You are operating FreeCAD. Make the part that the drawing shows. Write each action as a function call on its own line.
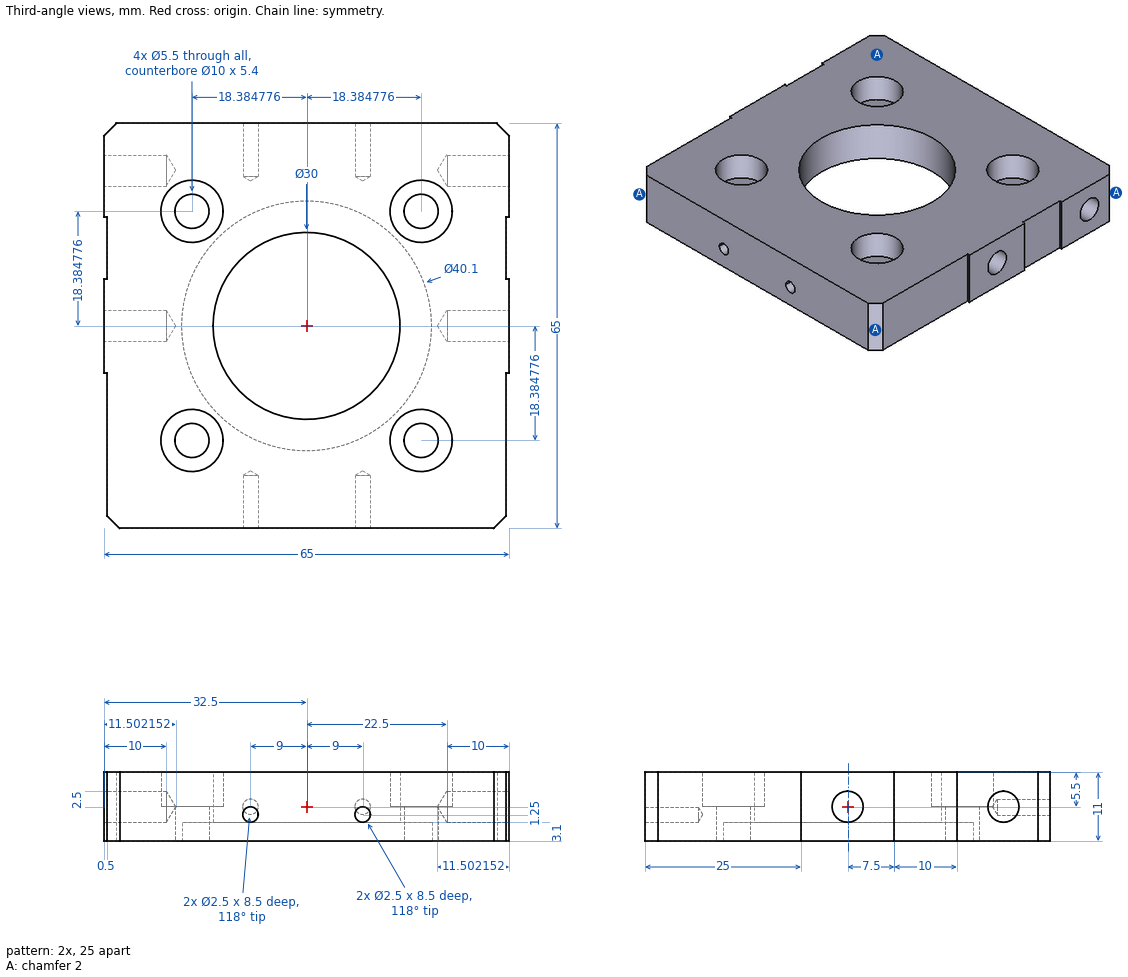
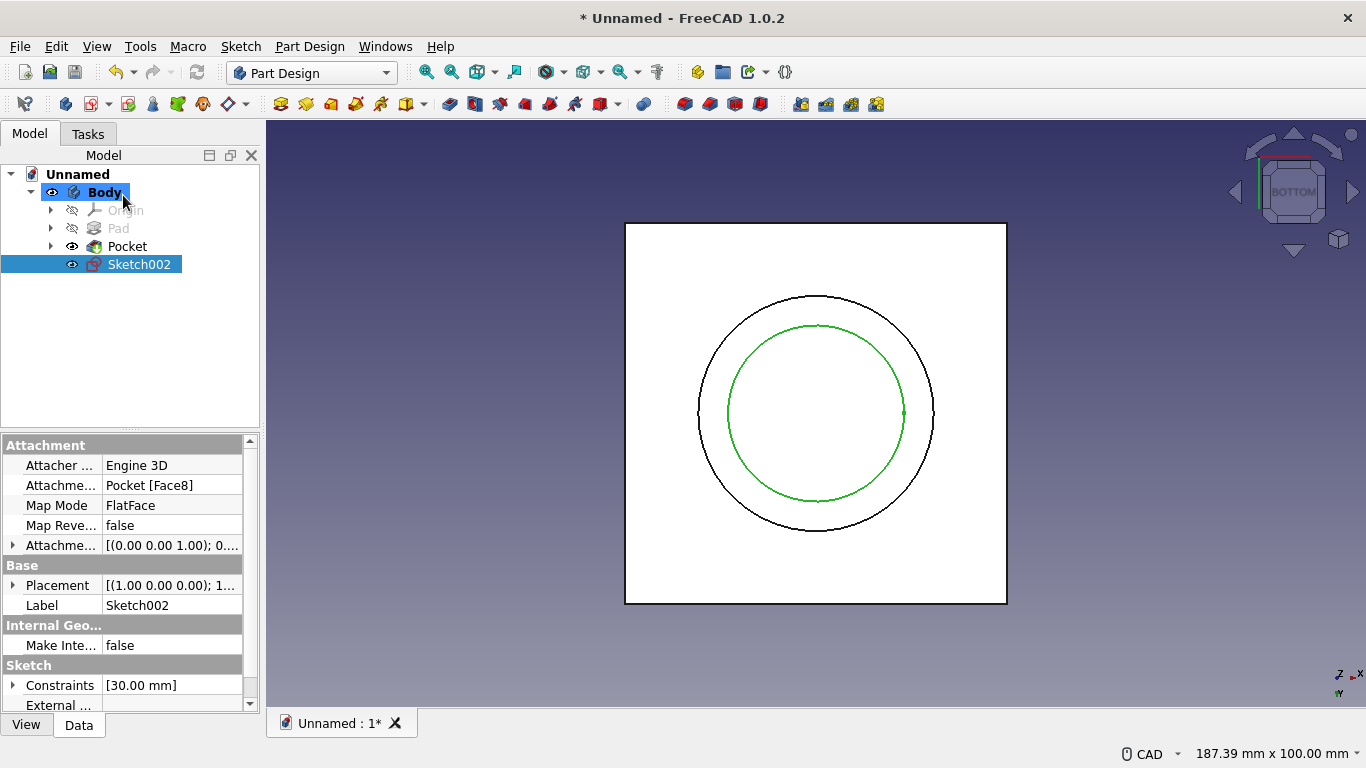
click(450, 104)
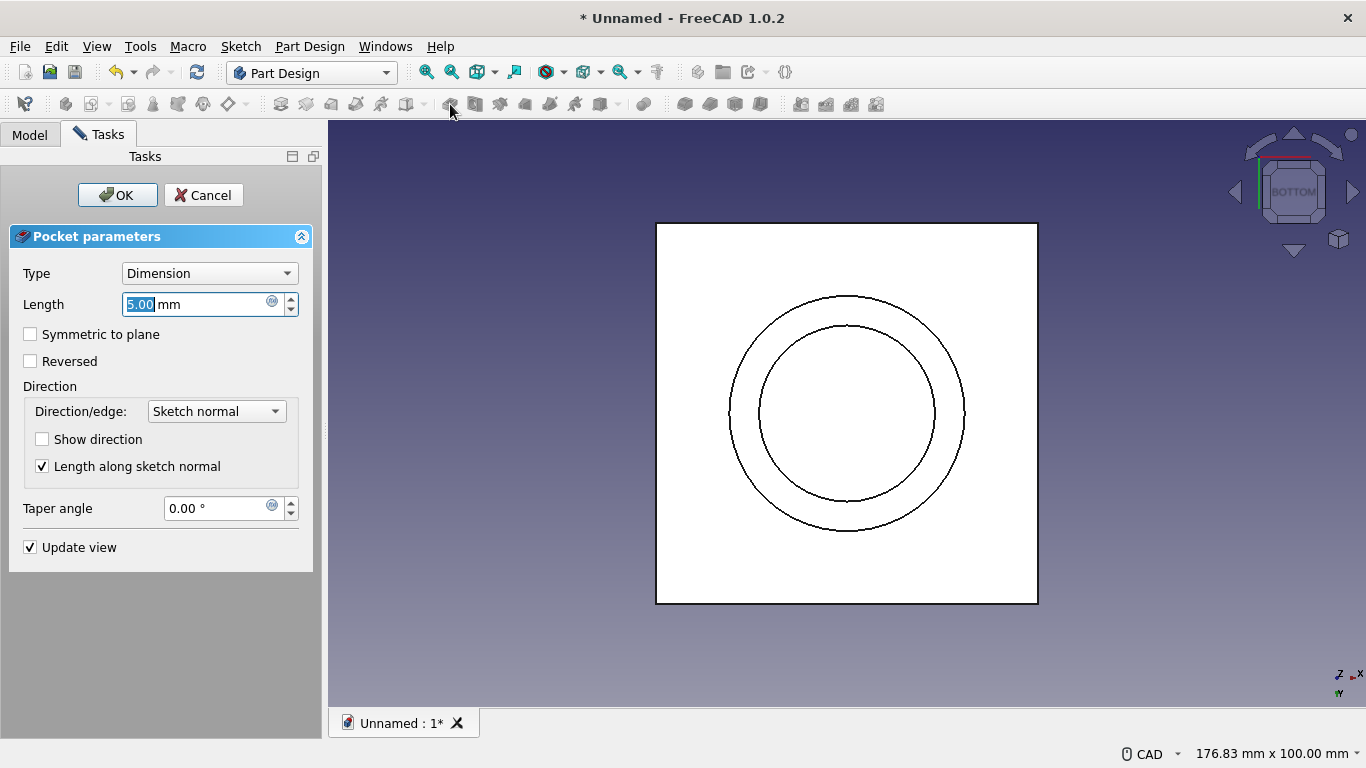
click(210, 274)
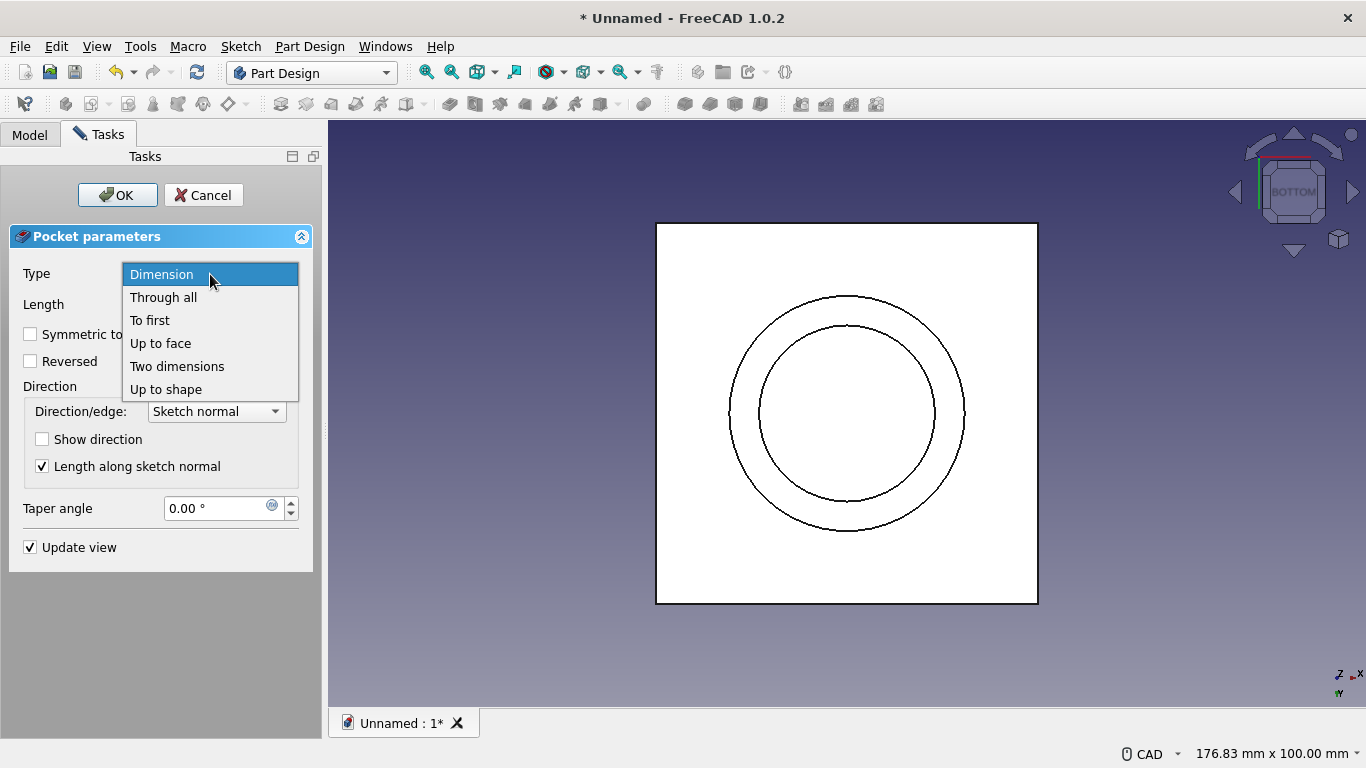
click(208, 298)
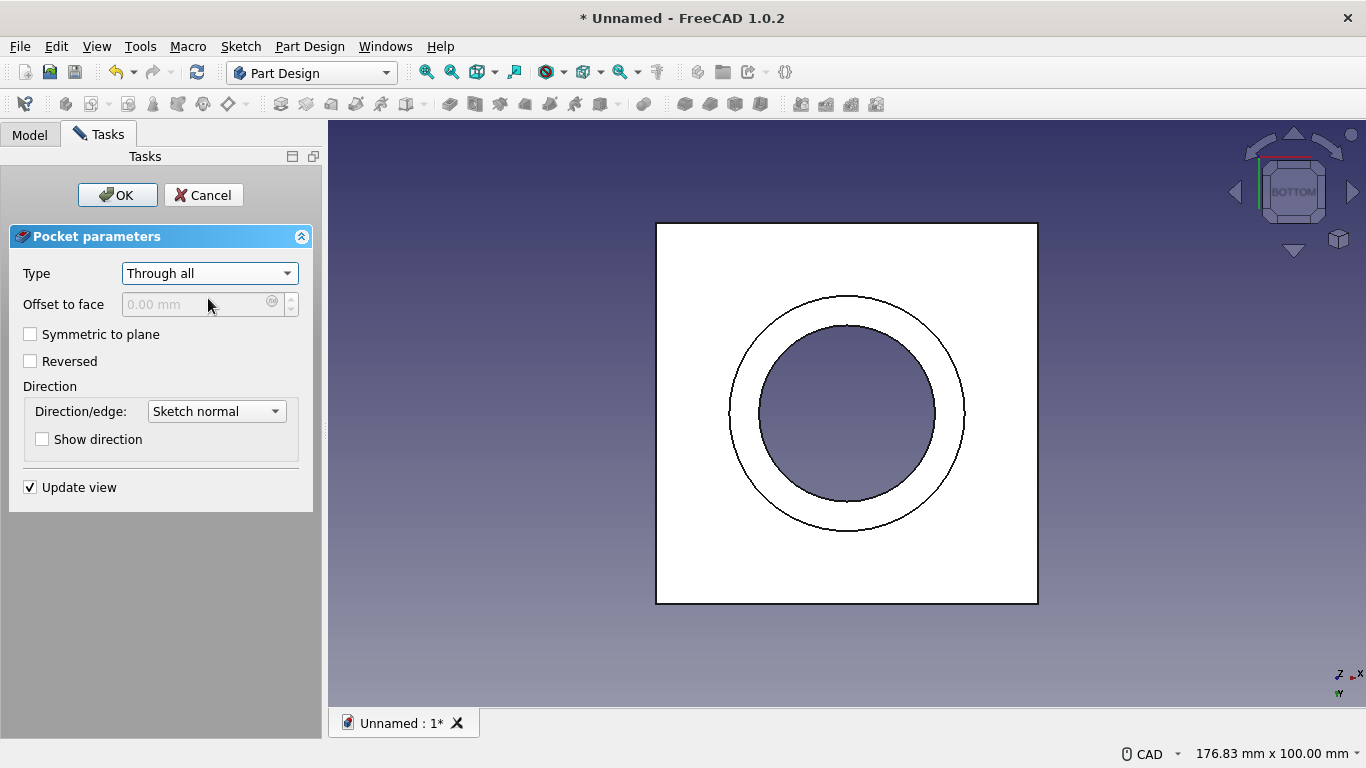
click(118, 195)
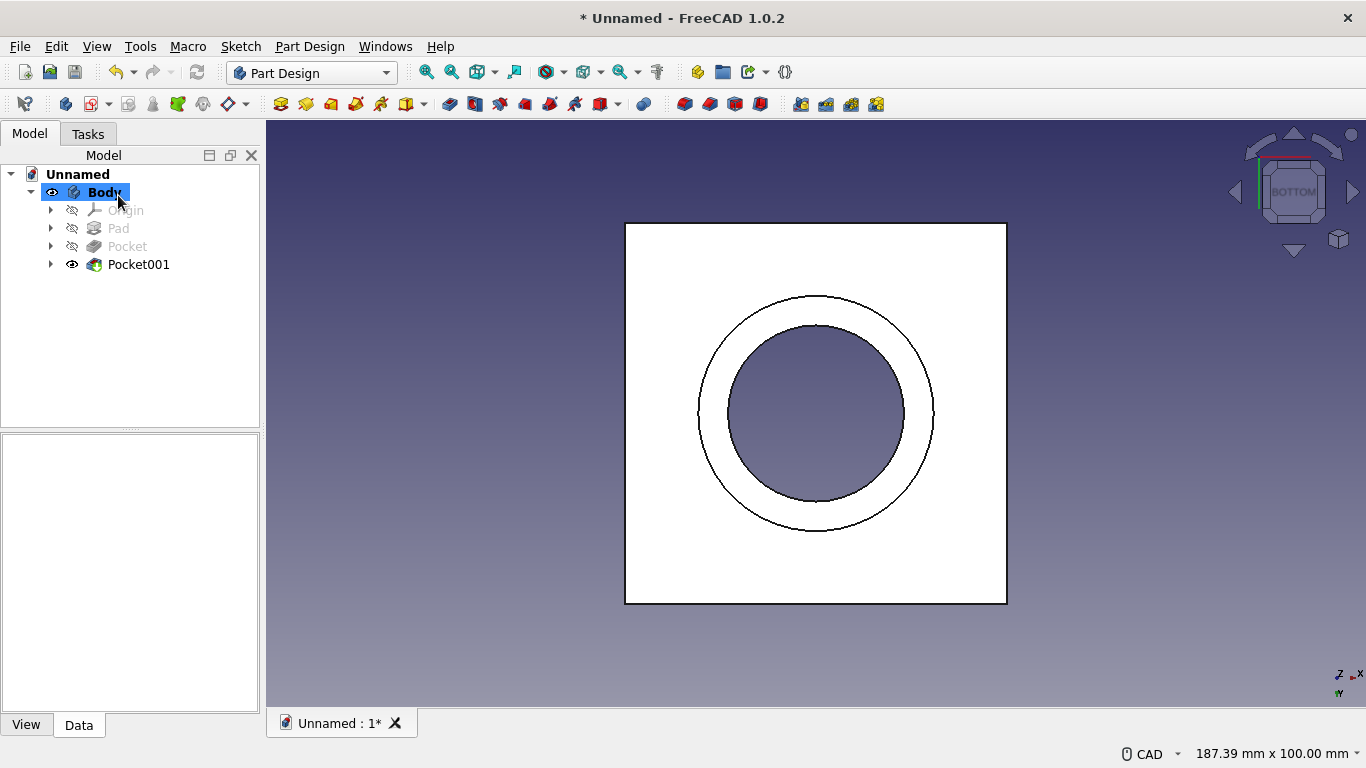
key(0)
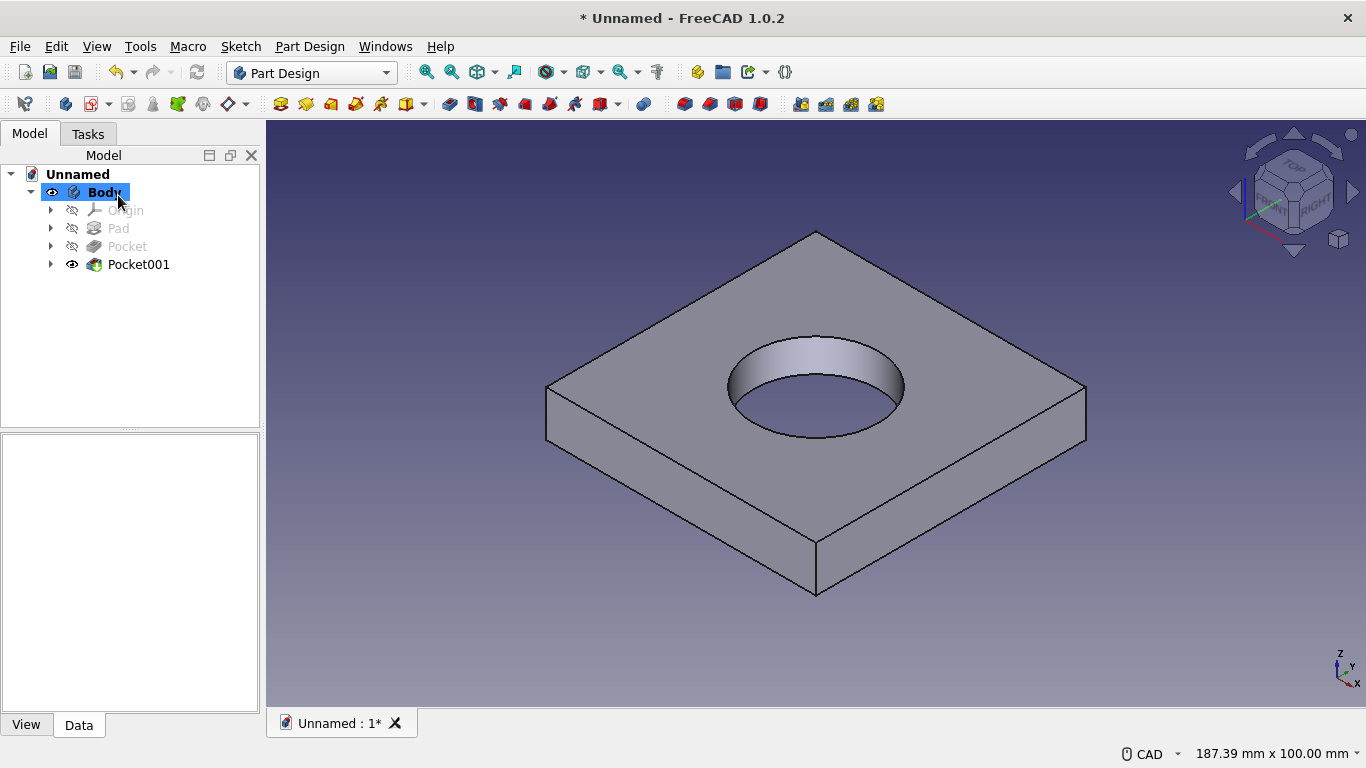
click(970, 386)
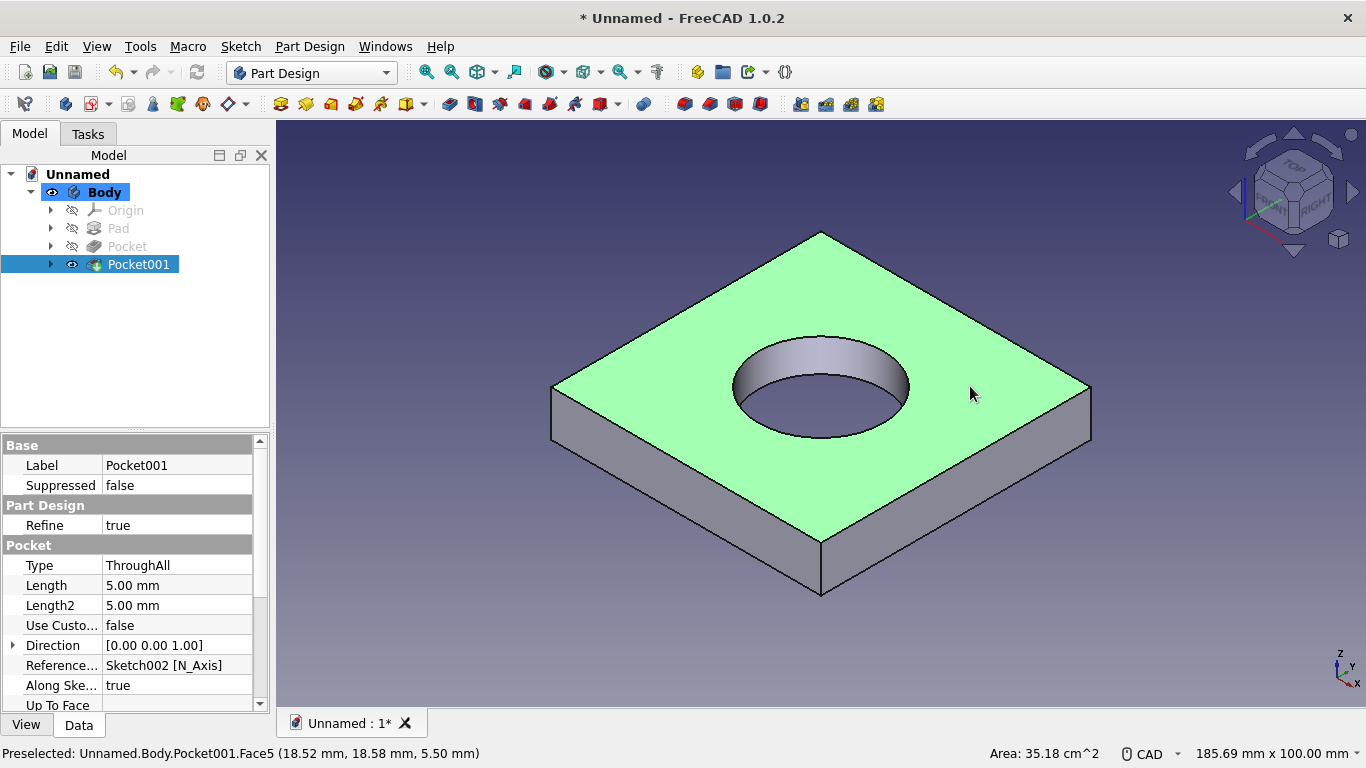
click(90, 104)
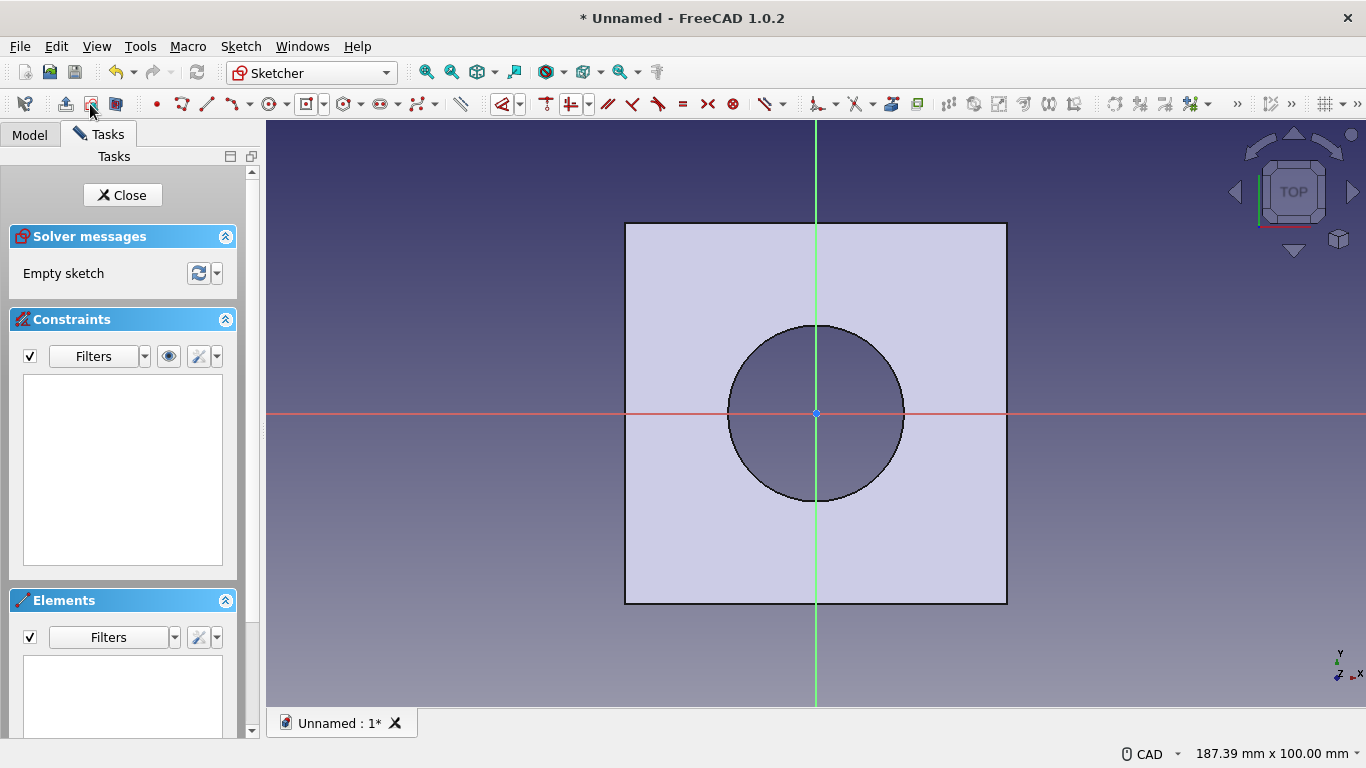
scroll(955, 413, up, 2)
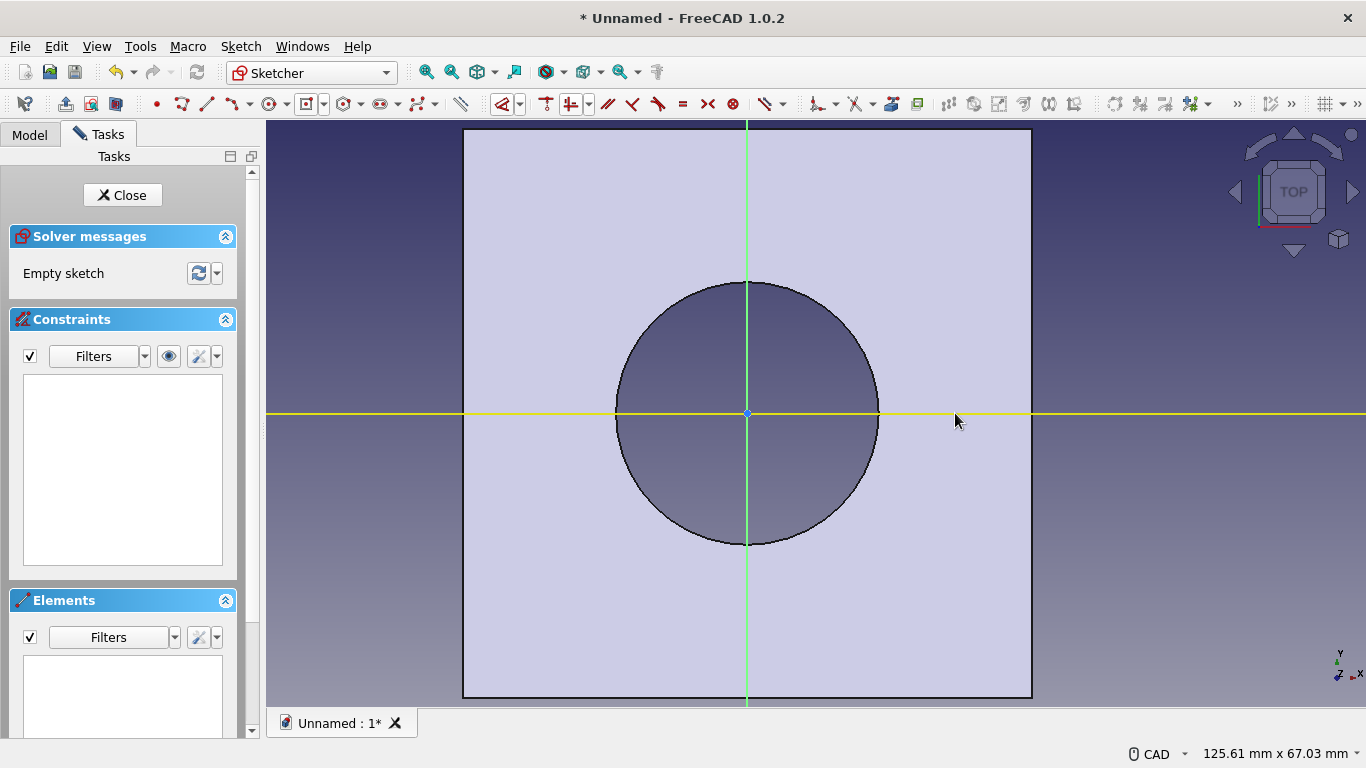
click(268, 104)